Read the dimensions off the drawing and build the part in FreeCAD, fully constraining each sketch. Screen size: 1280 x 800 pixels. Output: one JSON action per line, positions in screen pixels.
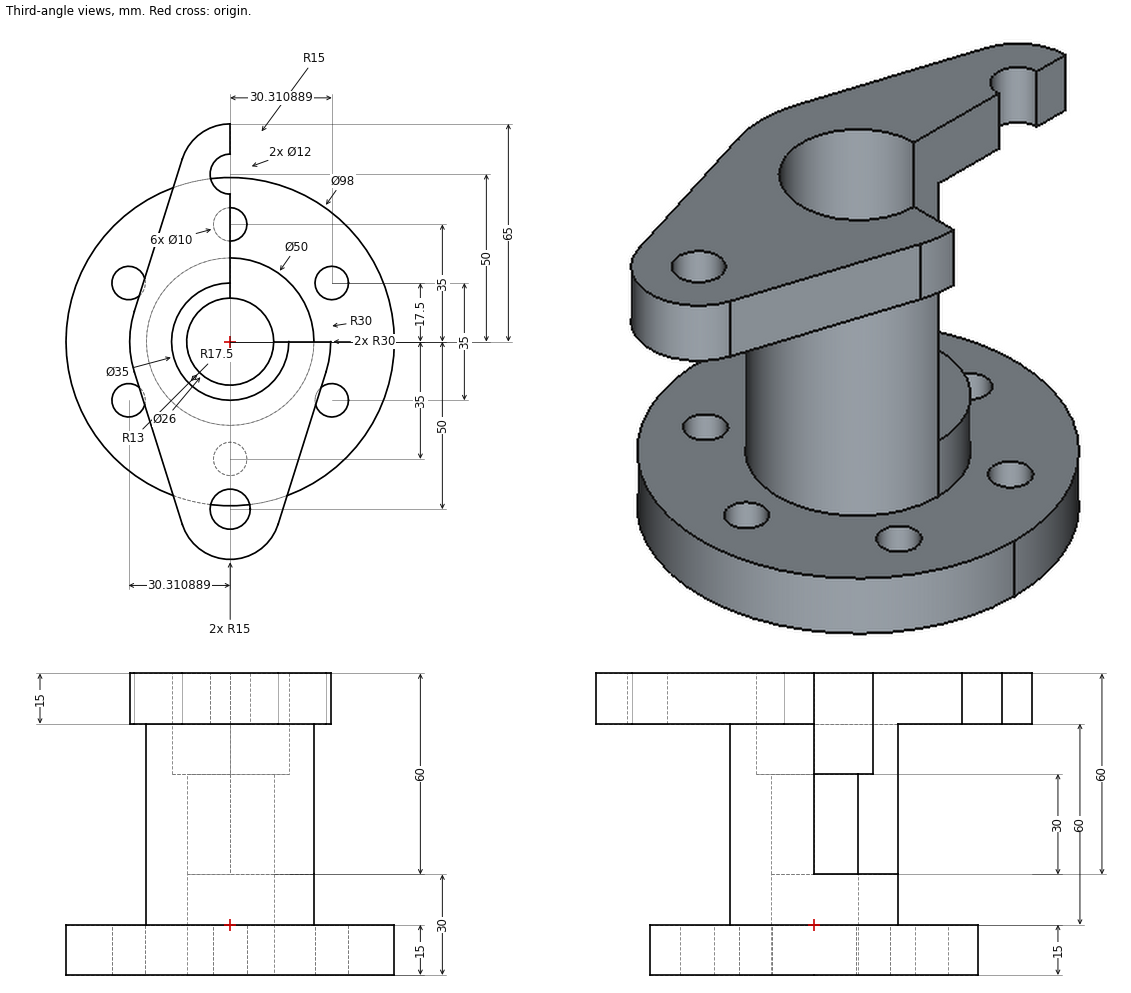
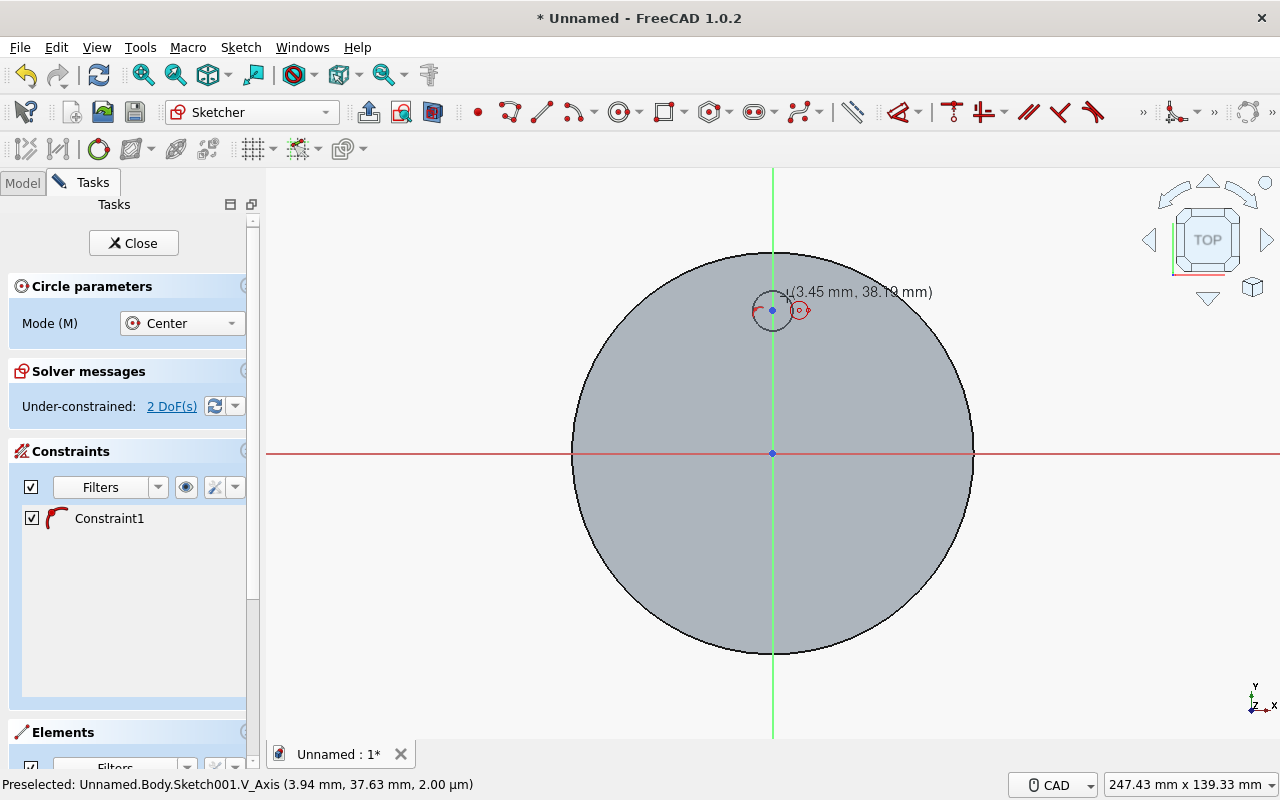
{"action": "left_click", "coordinate": [897, 382]}
{"action": "left_click", "coordinate": [912, 367]}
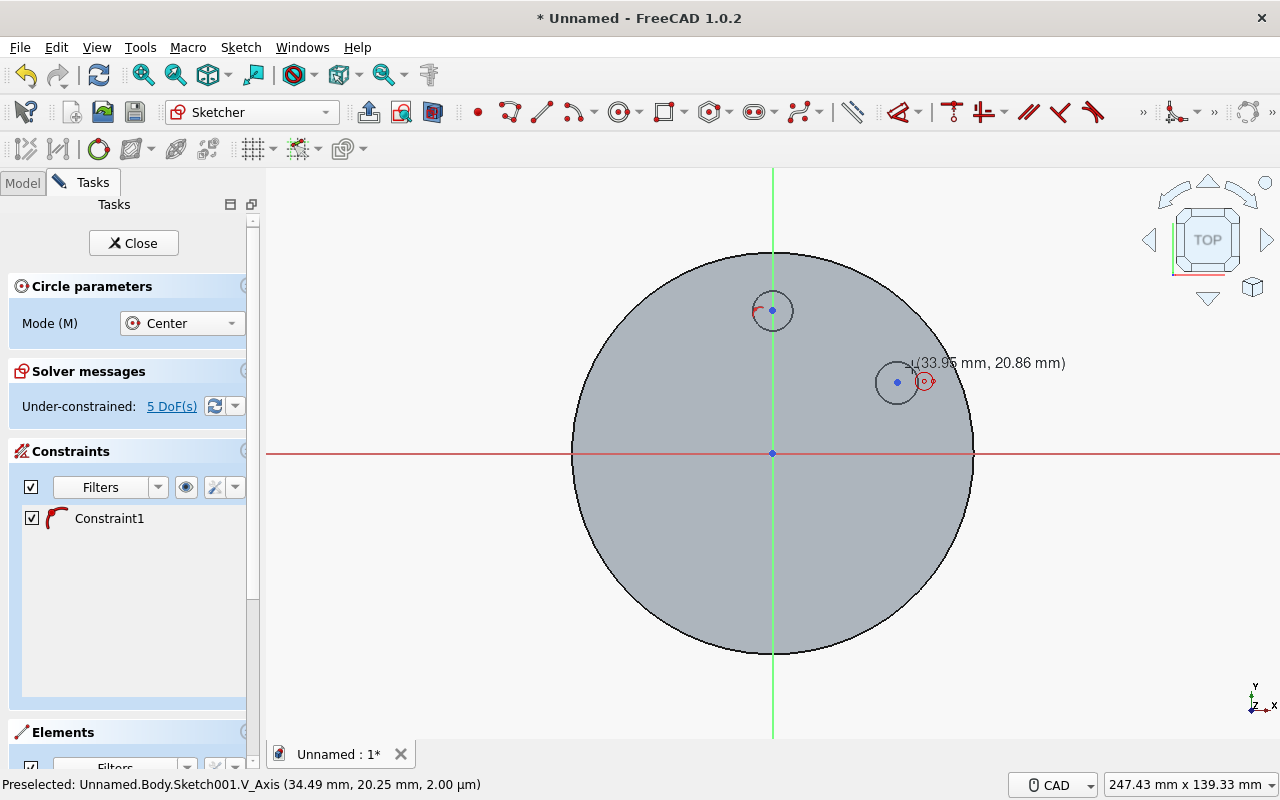
{"action": "left_click", "coordinate": [897, 525]}
{"action": "left_click", "coordinate": [912, 511]}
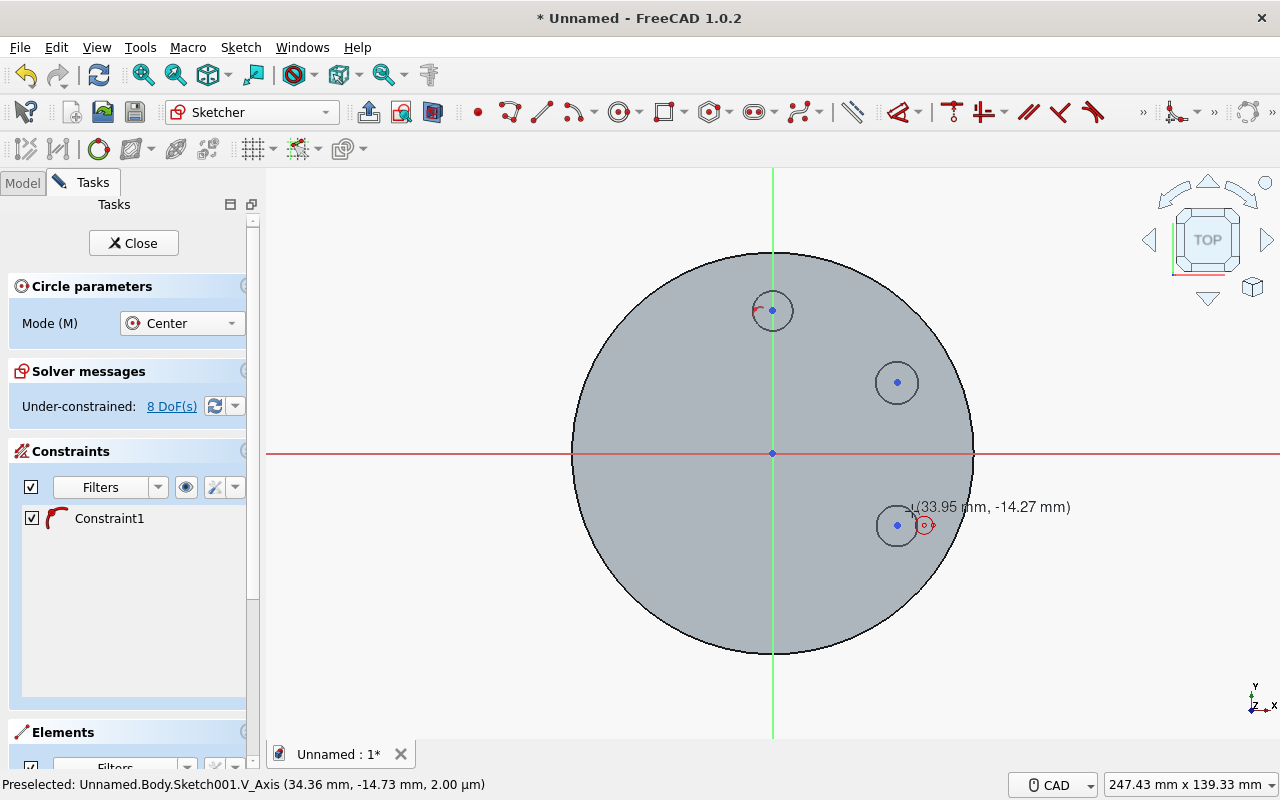
{"action": "left_click", "coordinate": [773, 597]}
{"action": "left_click", "coordinate": [787, 582]}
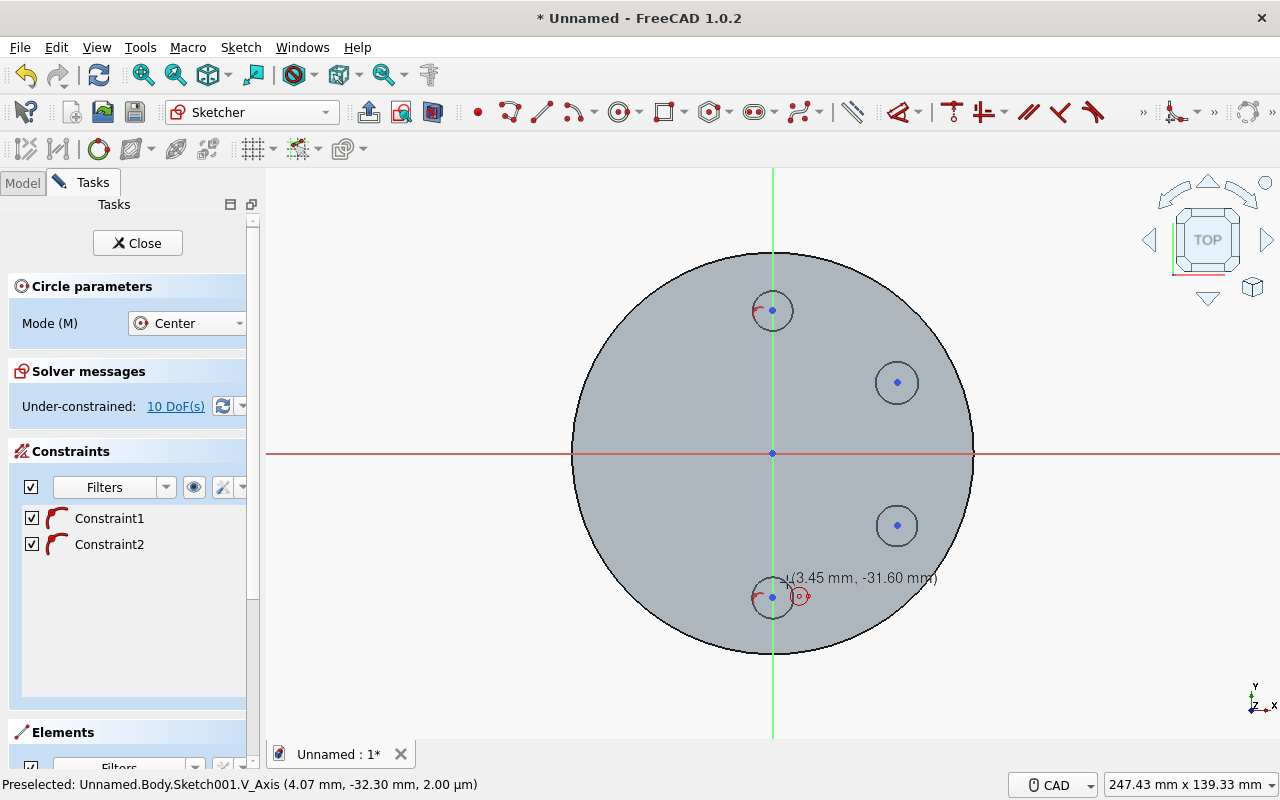
{"action": "left_click", "coordinate": [649, 525]}
{"action": "left_click", "coordinate": [663, 511]}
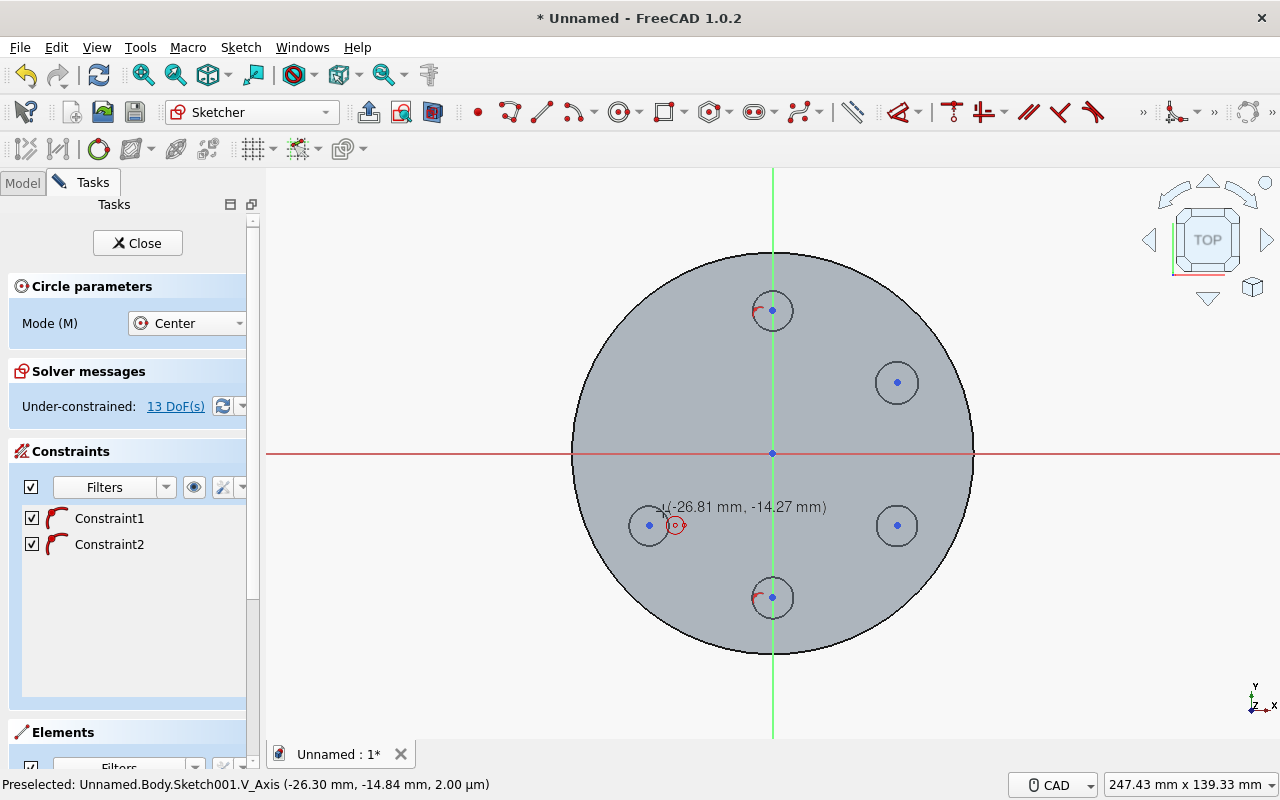
{"action": "left_click", "coordinate": [649, 382]}
{"action": "left_click", "coordinate": [663, 367]}
{"action": "key", "text": "Escape"}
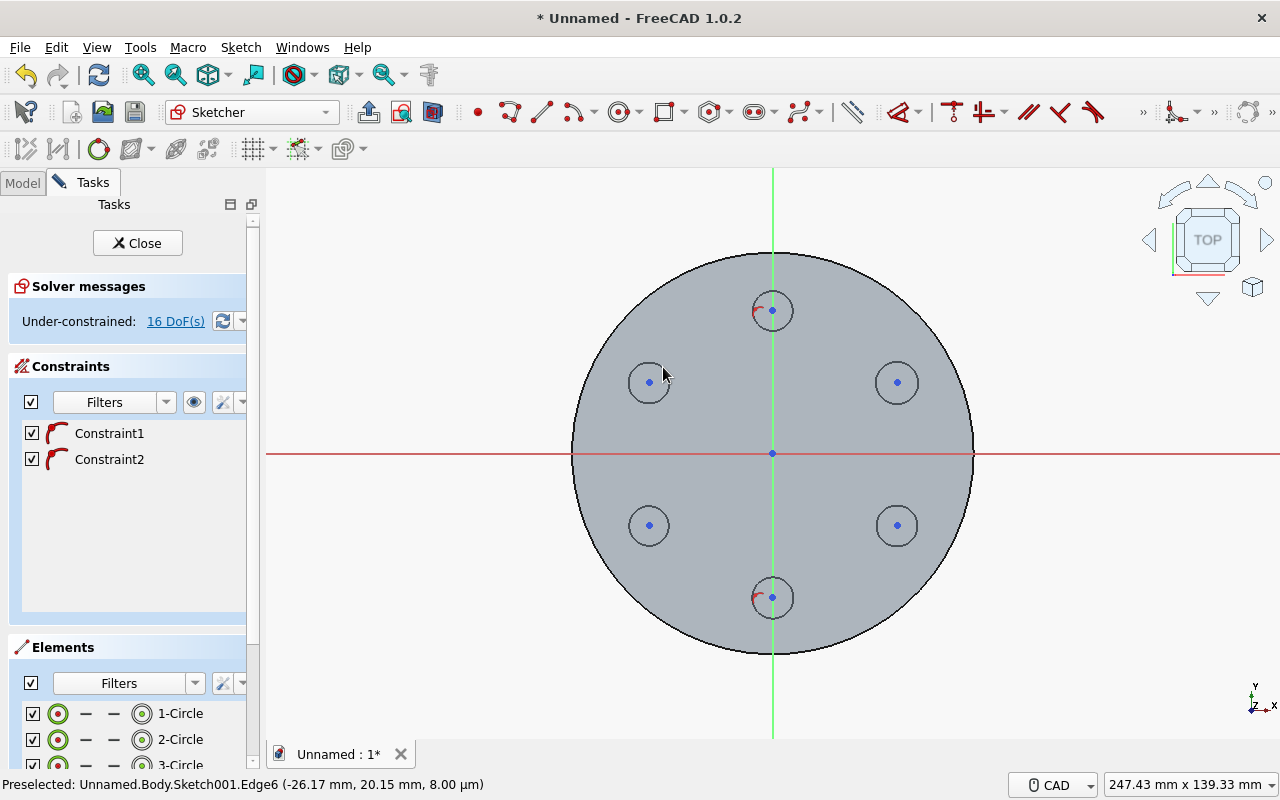
{"action": "left_click", "coordinate": [787, 297]}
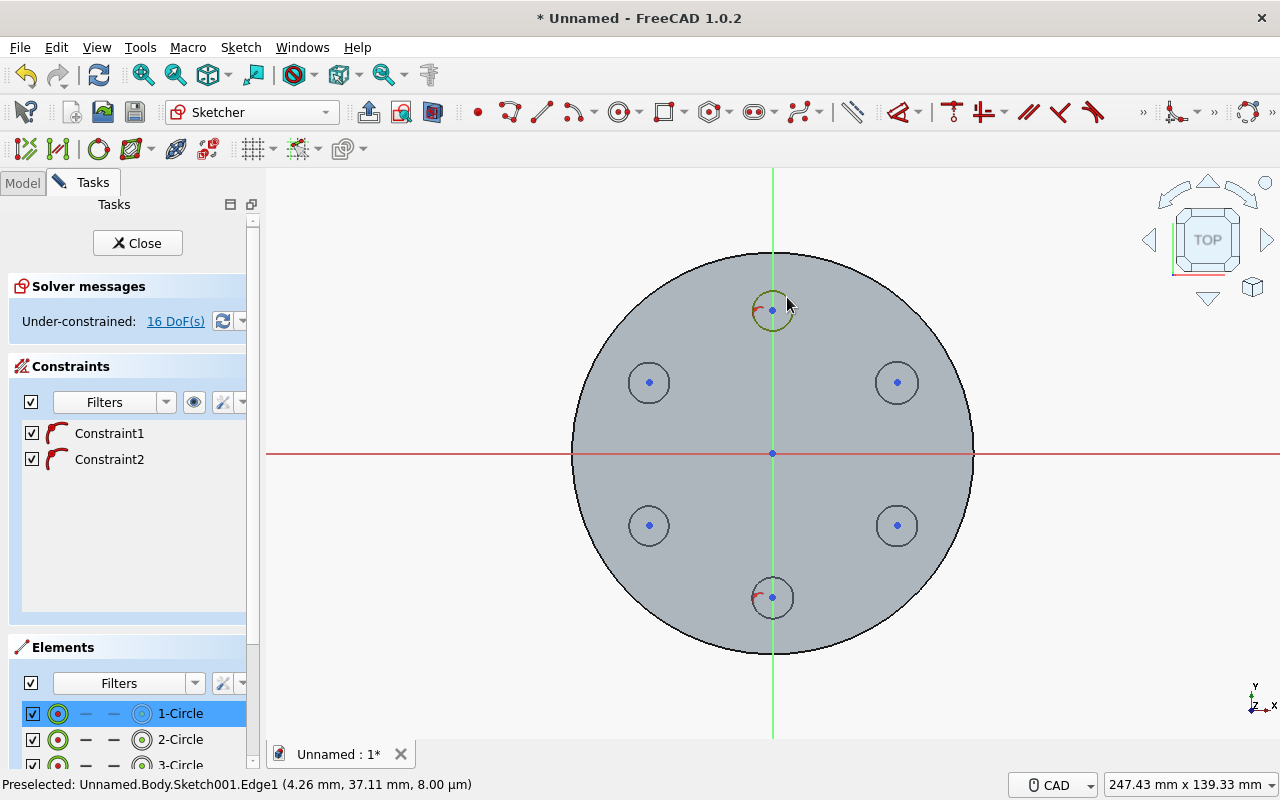
{"action": "left_click", "coordinate": [912, 368]}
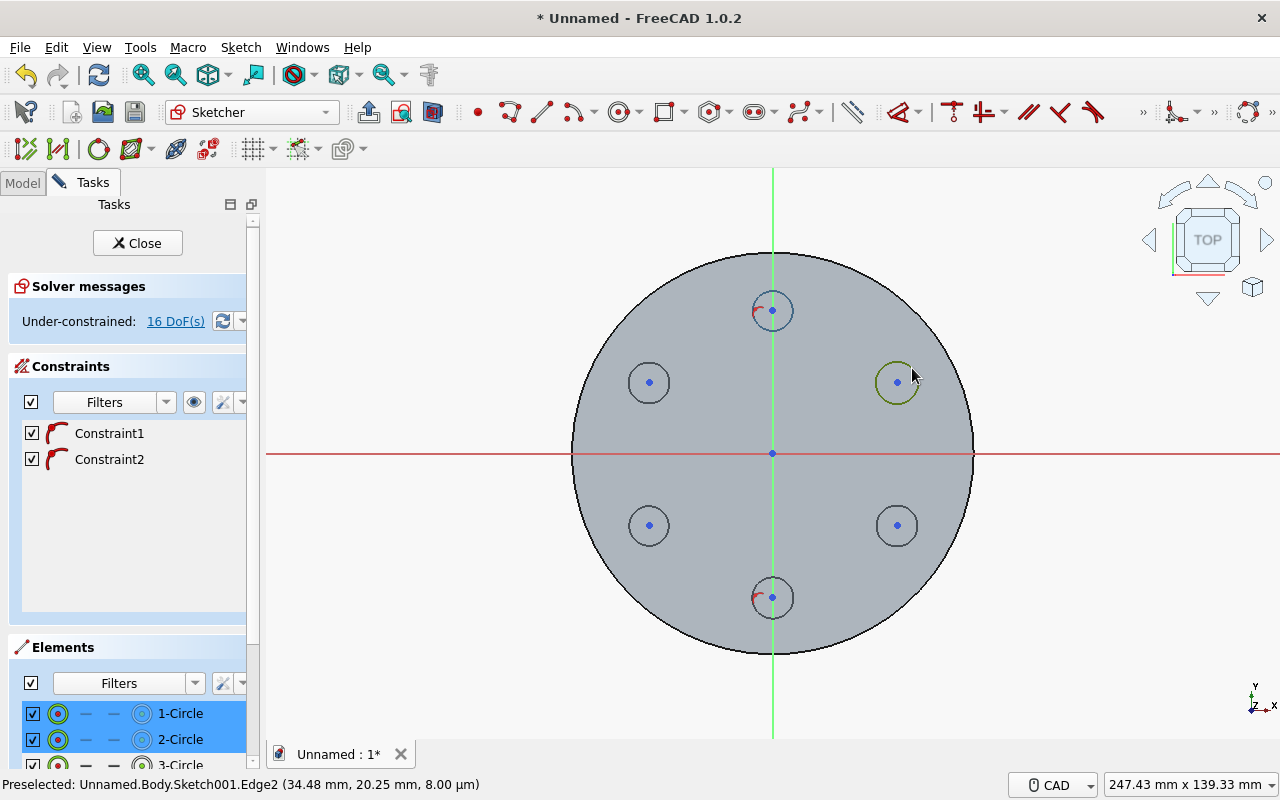
{"action": "left_click", "coordinate": [911, 511]}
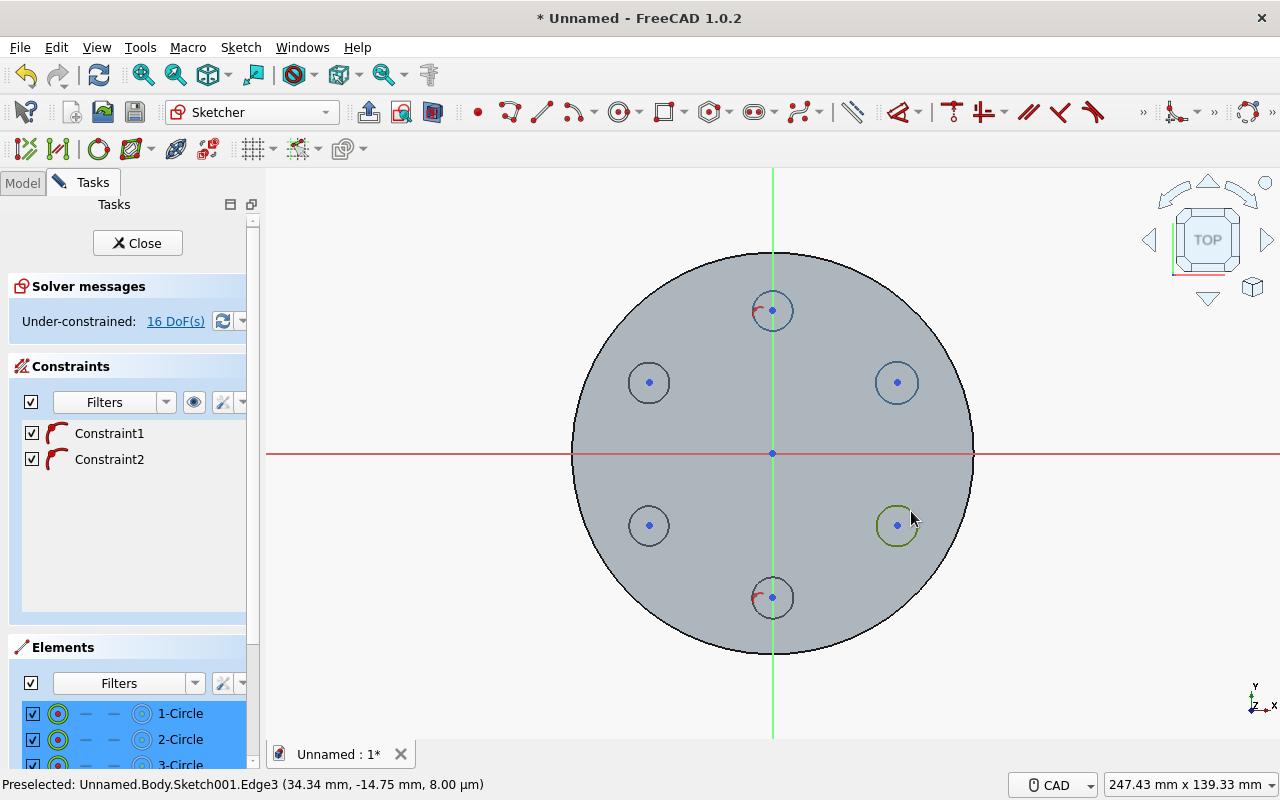
{"action": "left_click", "coordinate": [787, 583]}